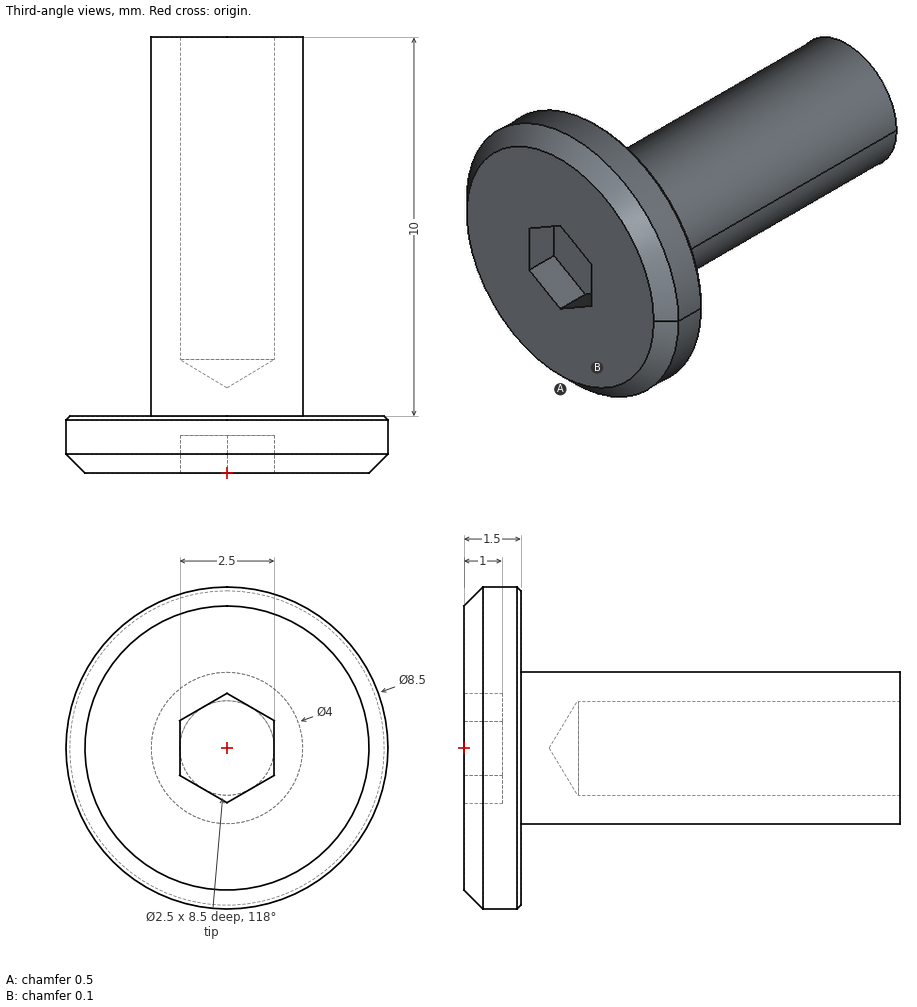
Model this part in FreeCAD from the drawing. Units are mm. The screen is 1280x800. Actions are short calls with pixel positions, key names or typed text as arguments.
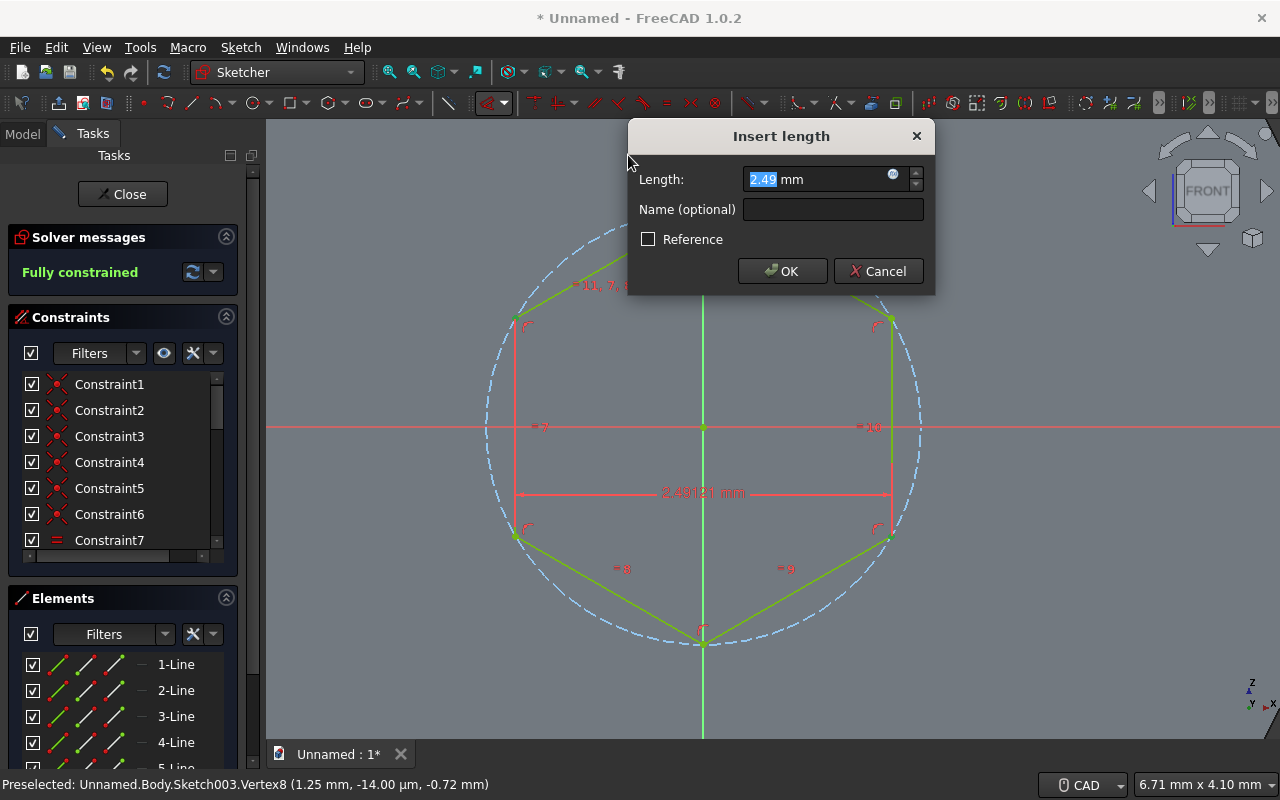
text(2.5)
key(Return)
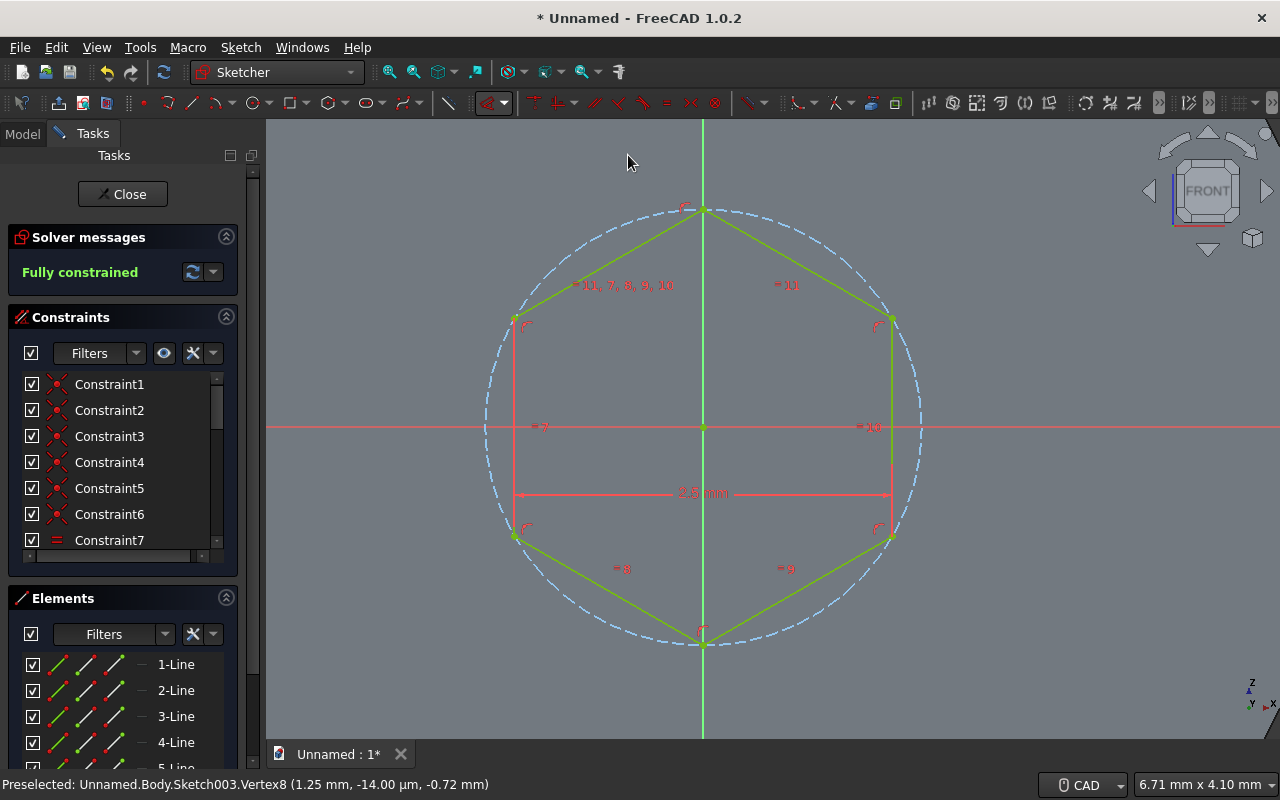
click(123, 194)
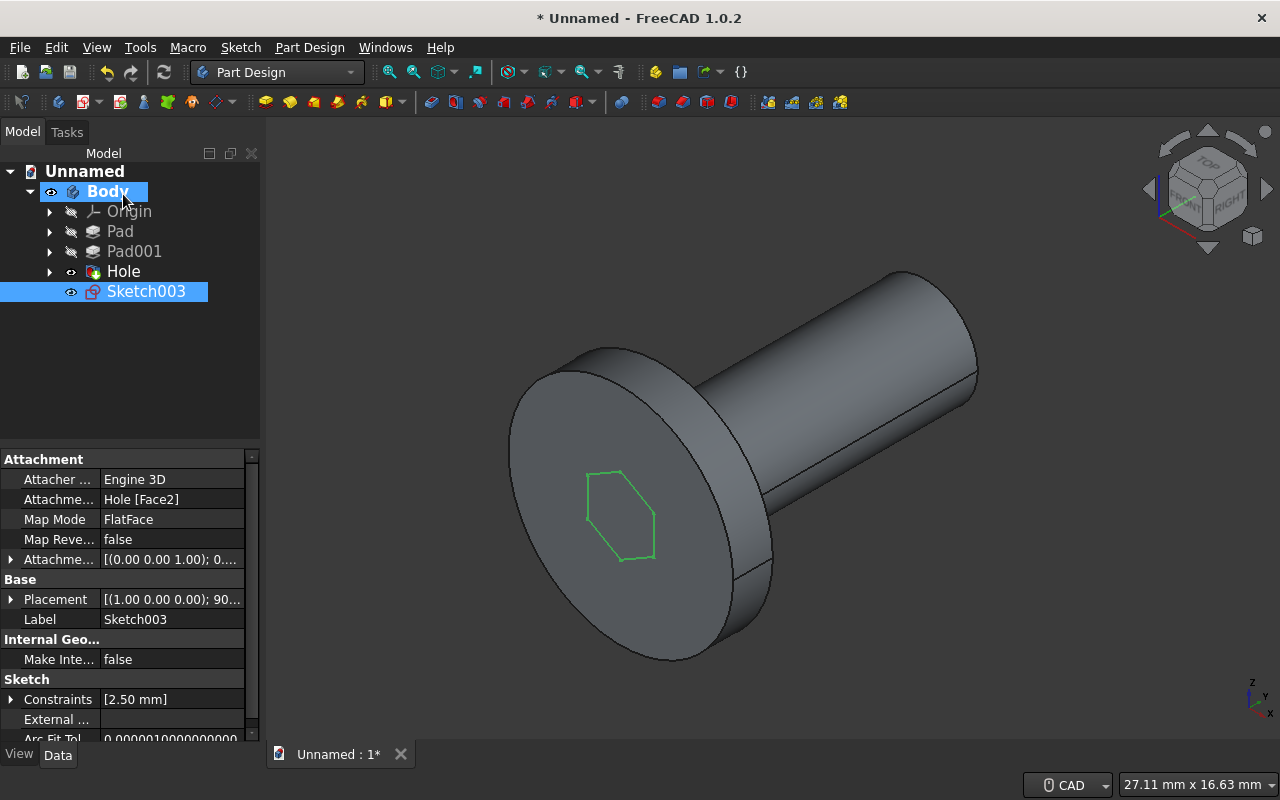
click(432, 102)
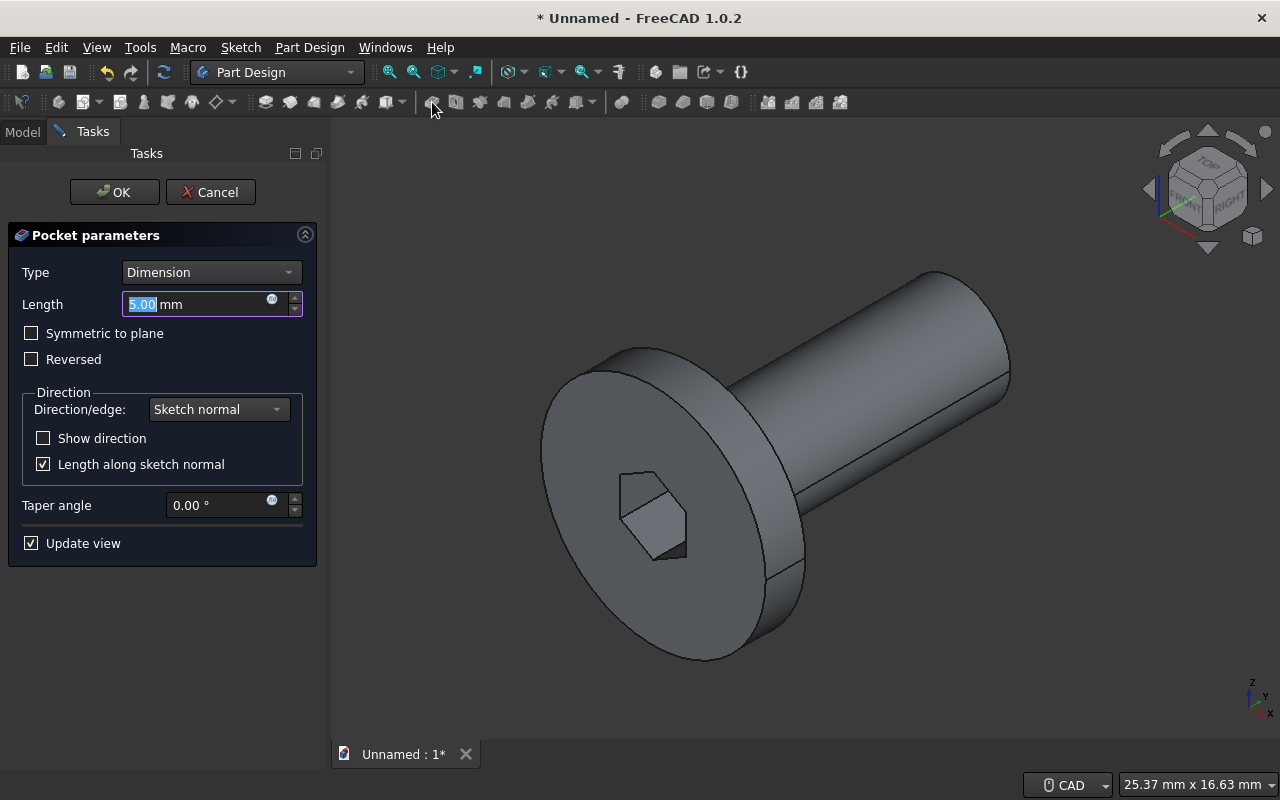
text(1)
key(Tab)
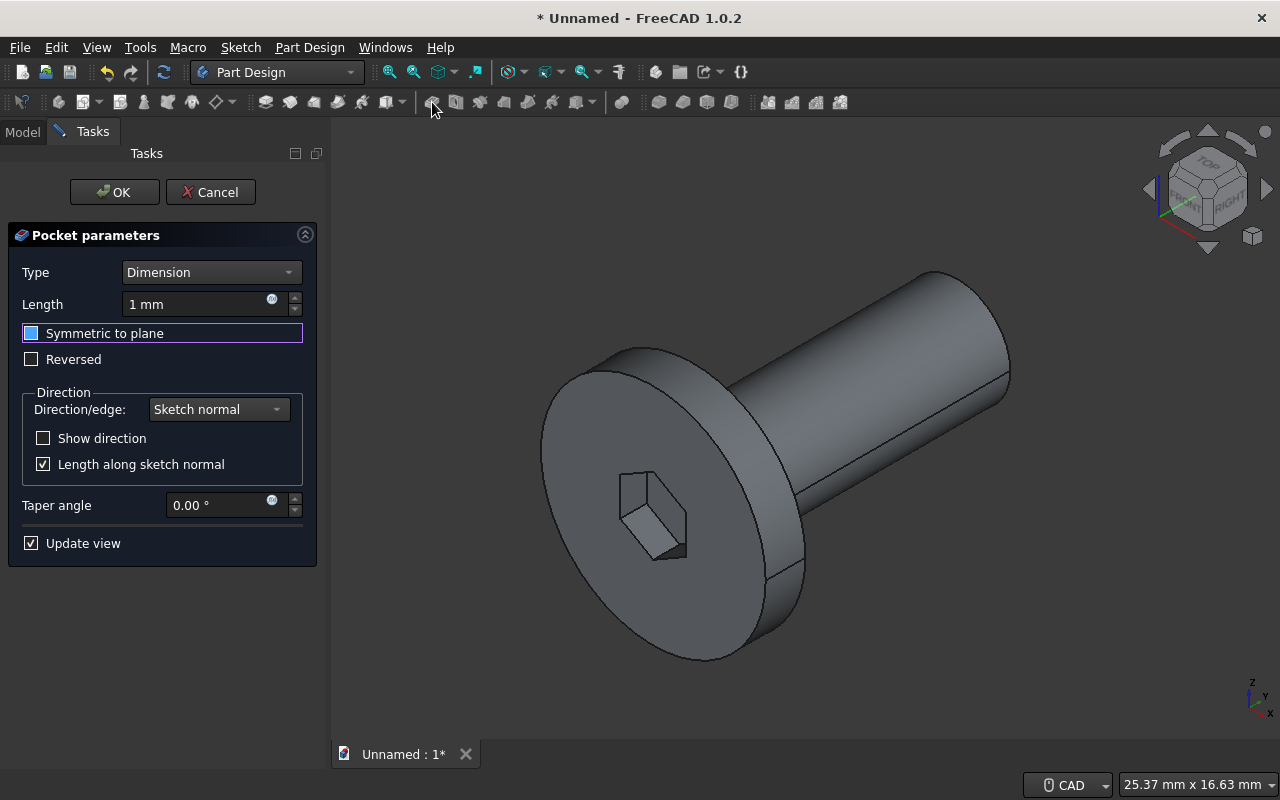
click(115, 192)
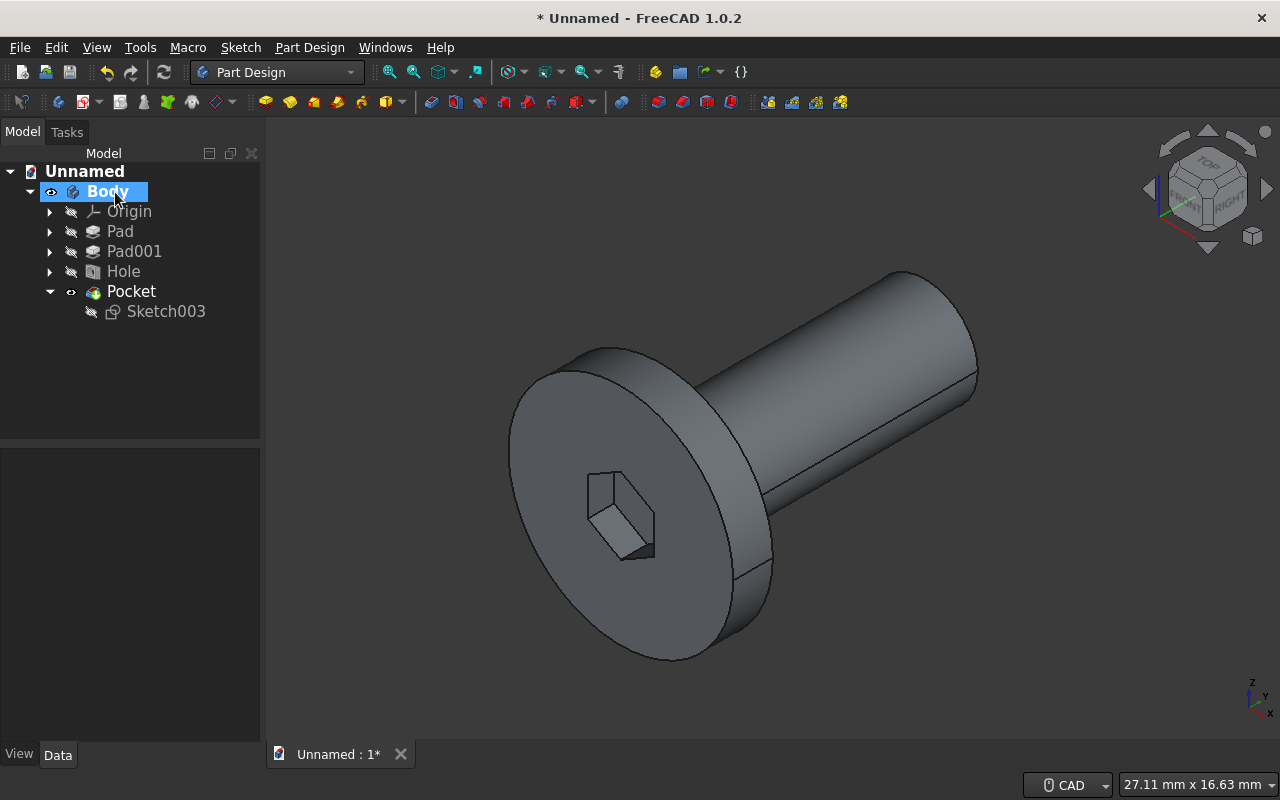
click(586, 371)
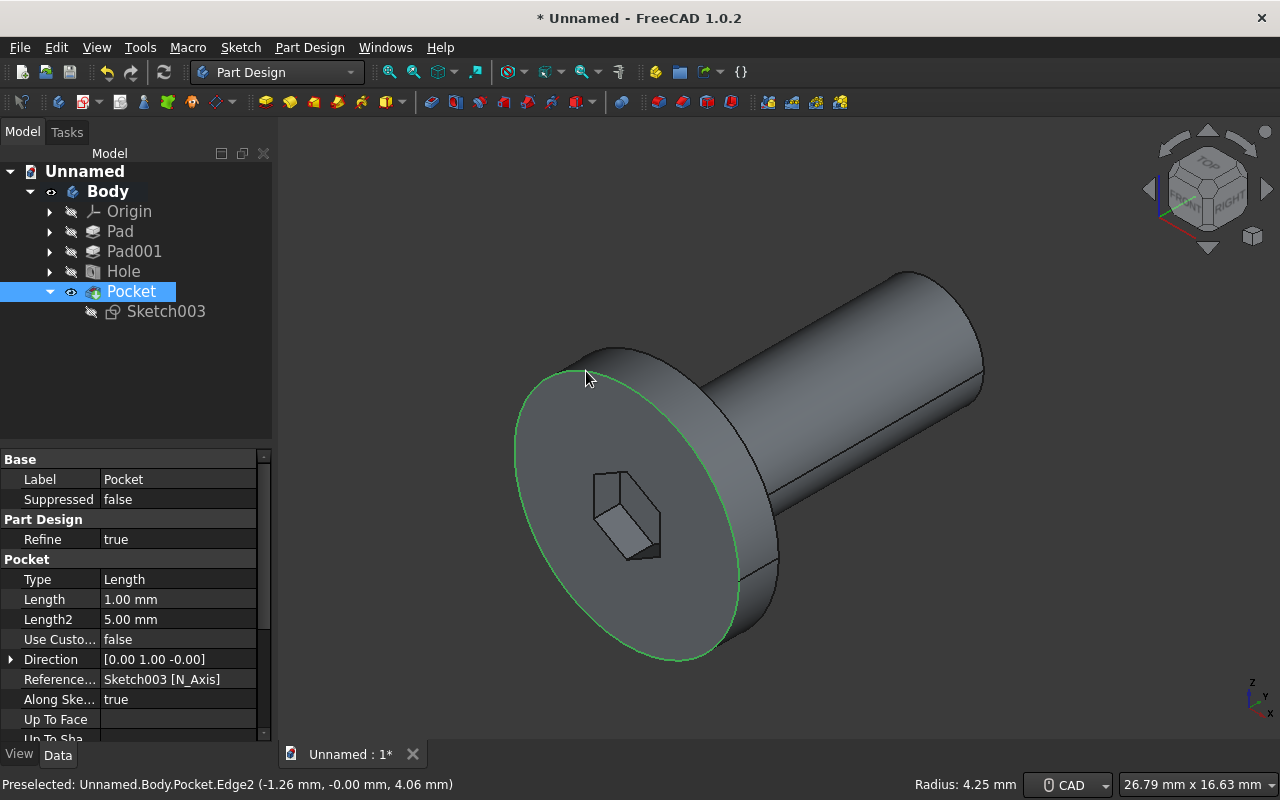
click(684, 102)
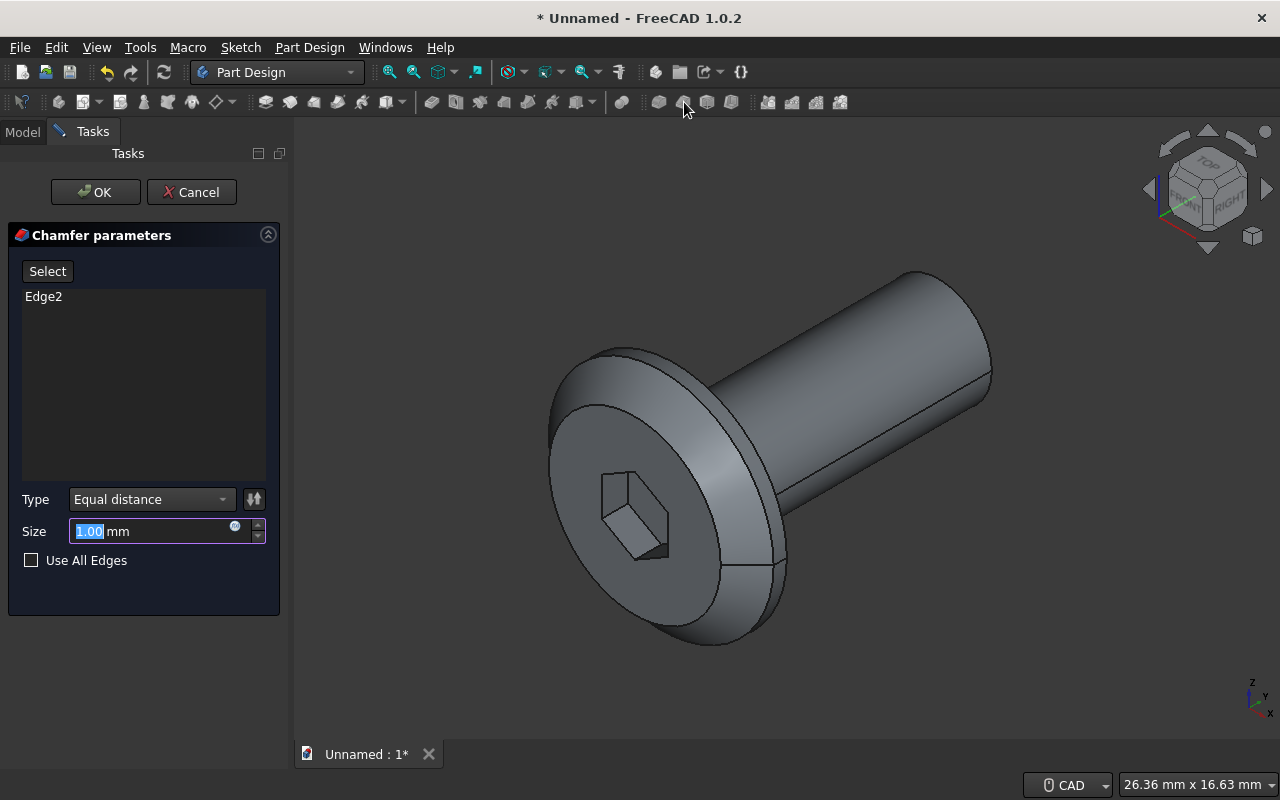
text(0.5)
key(Tab)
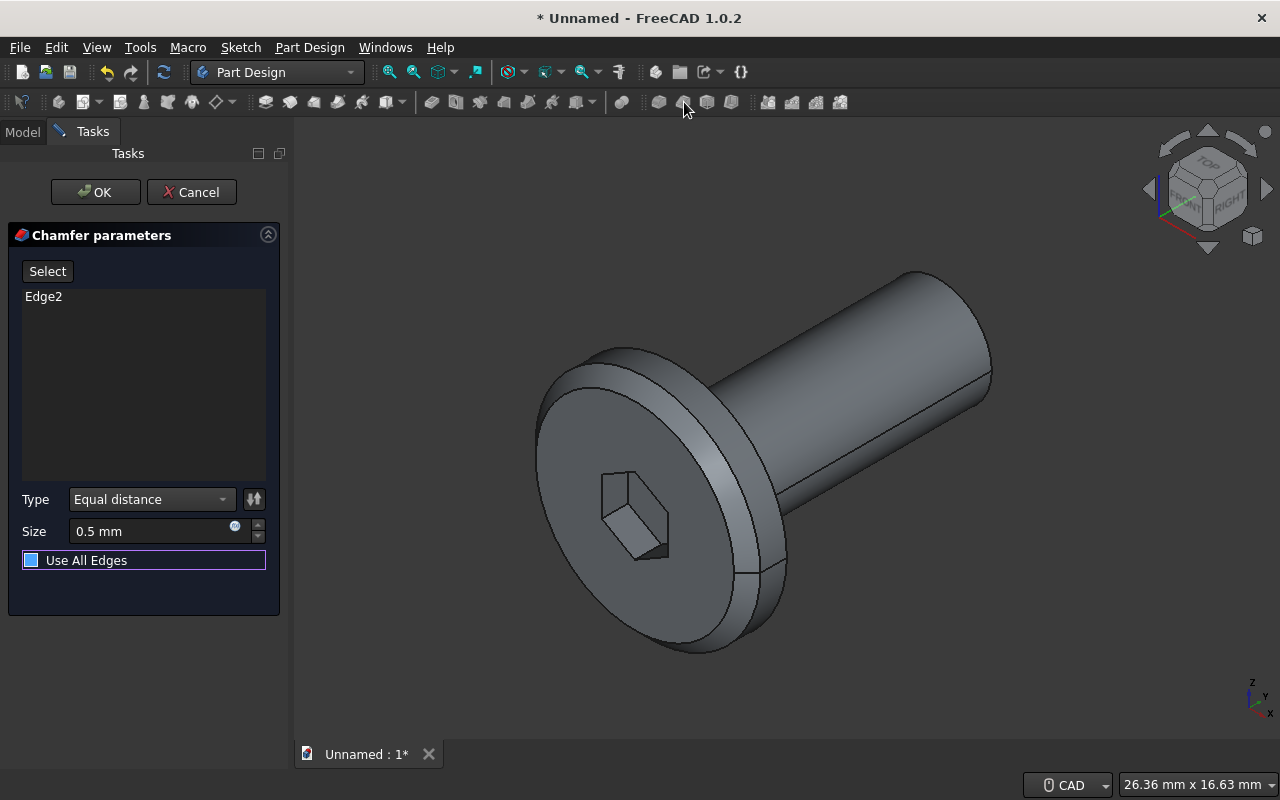
click(96, 192)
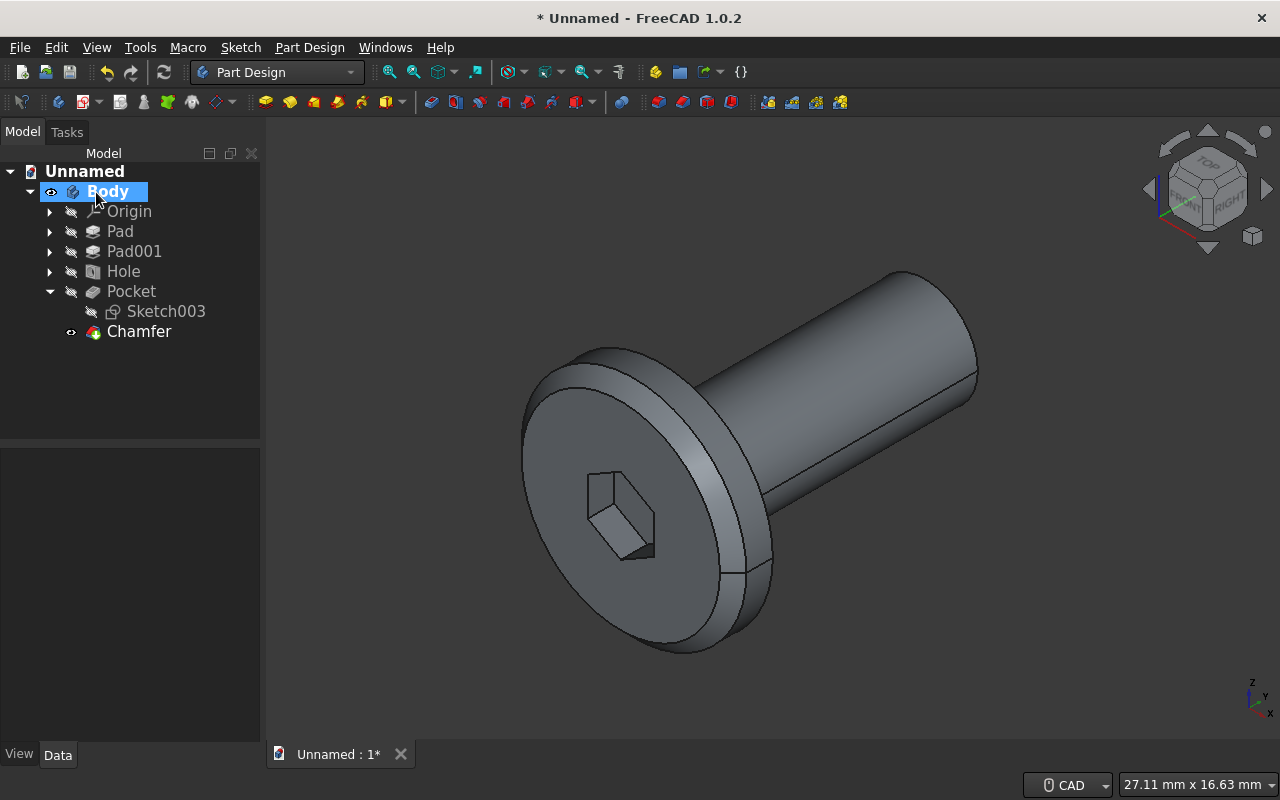
key(2)